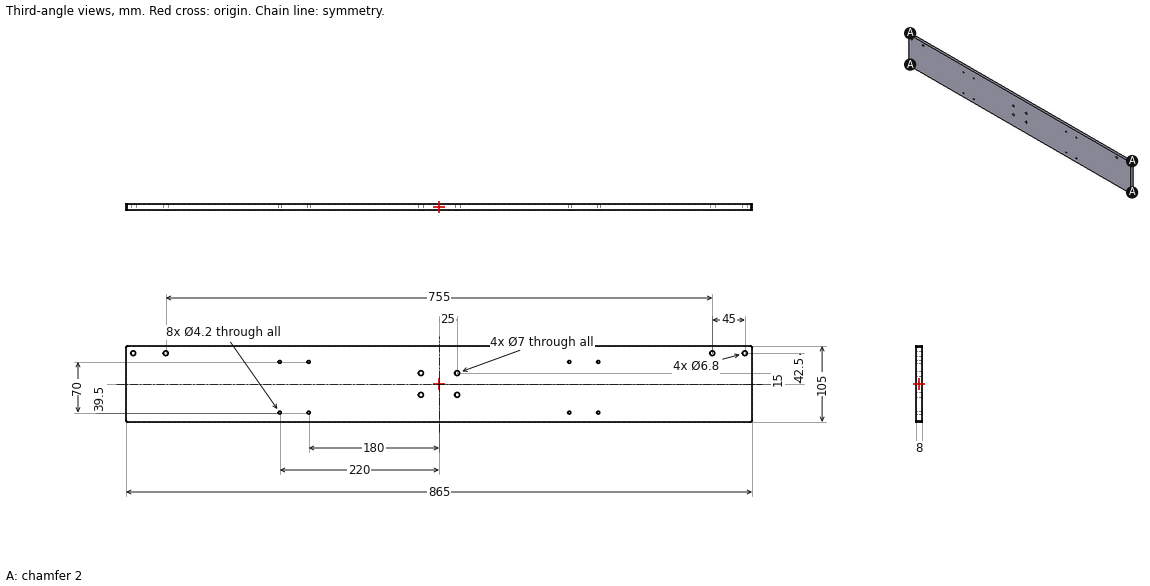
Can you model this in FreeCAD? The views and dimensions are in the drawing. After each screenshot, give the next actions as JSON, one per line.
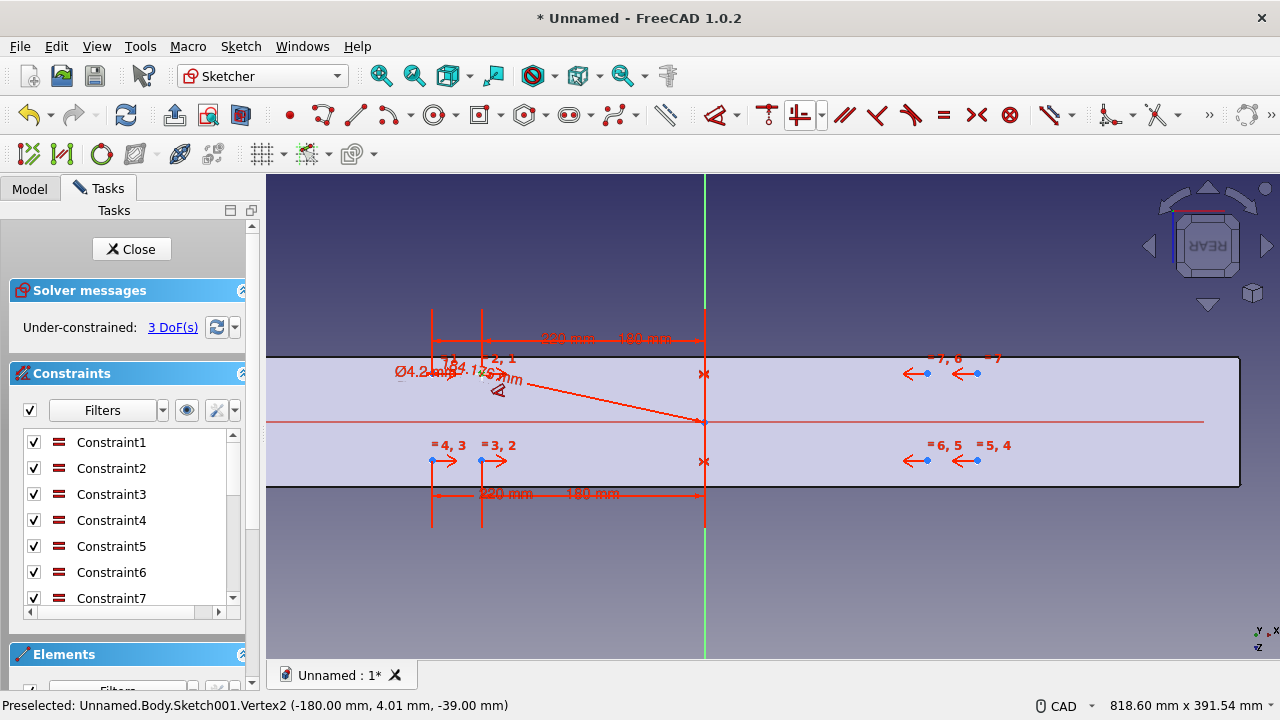
{"action": "left_click", "coordinate": [482, 461]}
{"action": "left_click", "coordinate": [448, 397]}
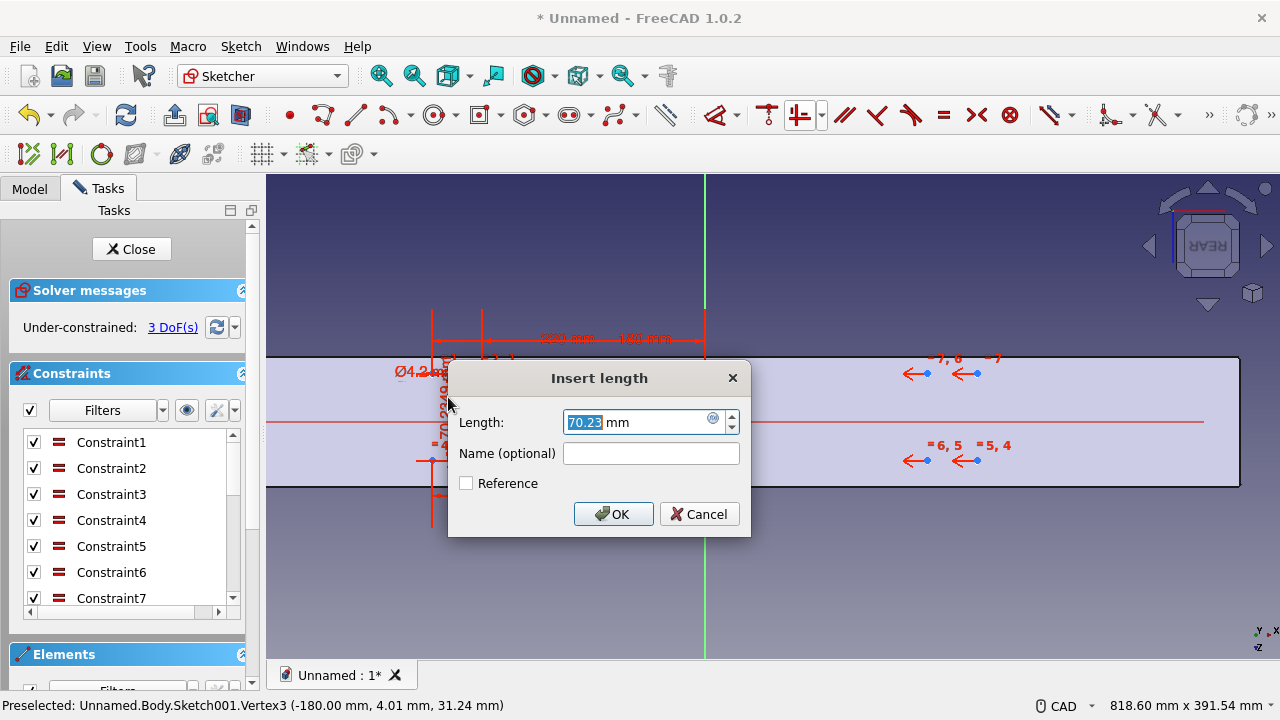
{"action": "type", "text": "70"}
{"action": "key", "text": "Return"}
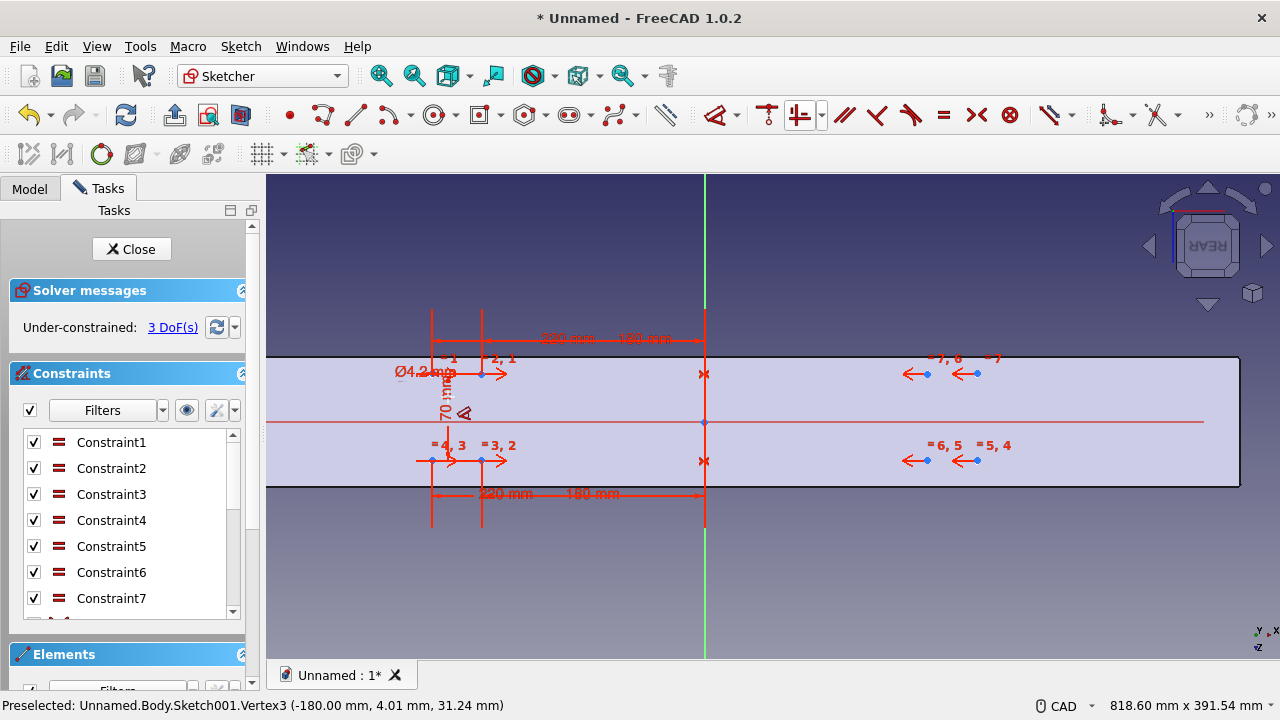
{"action": "left_click", "coordinate": [432, 374]}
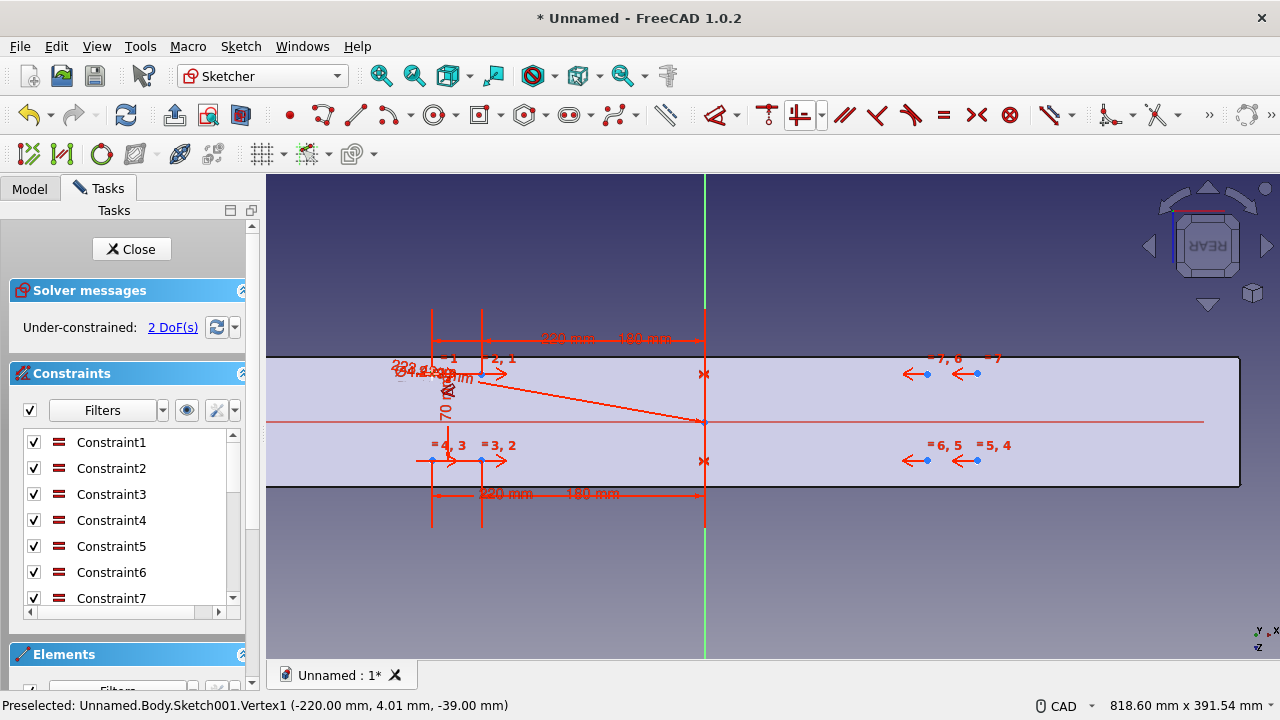
{"action": "left_click", "coordinate": [482, 461]}
{"action": "left_click", "coordinate": [398, 437]}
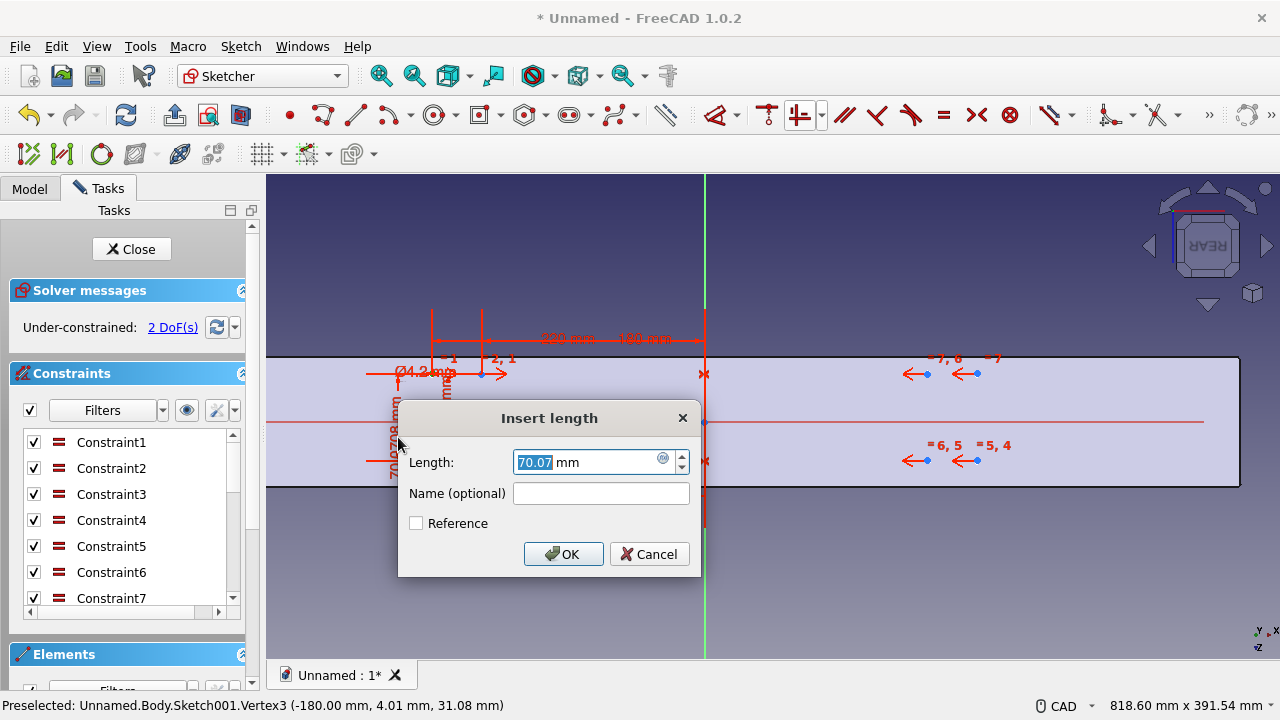
{"action": "type", "text": "70"}
{"action": "key", "text": "Return"}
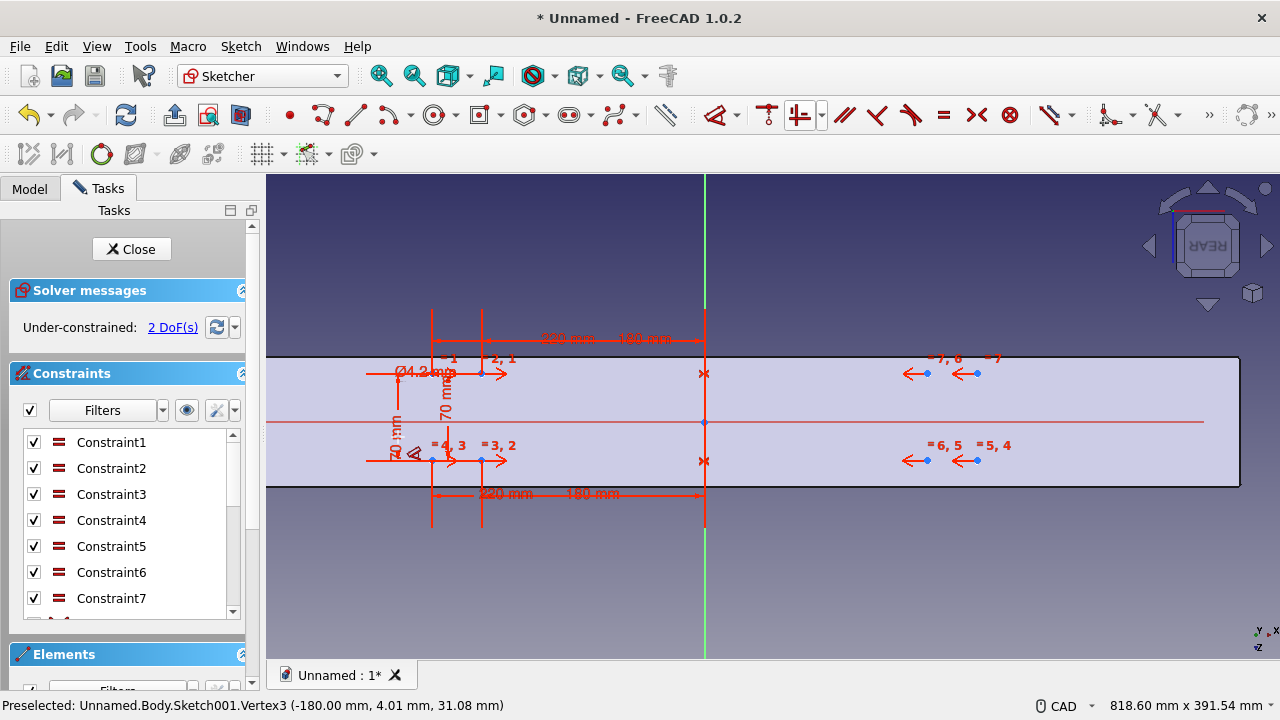
{"action": "left_click", "coordinate": [432, 374]}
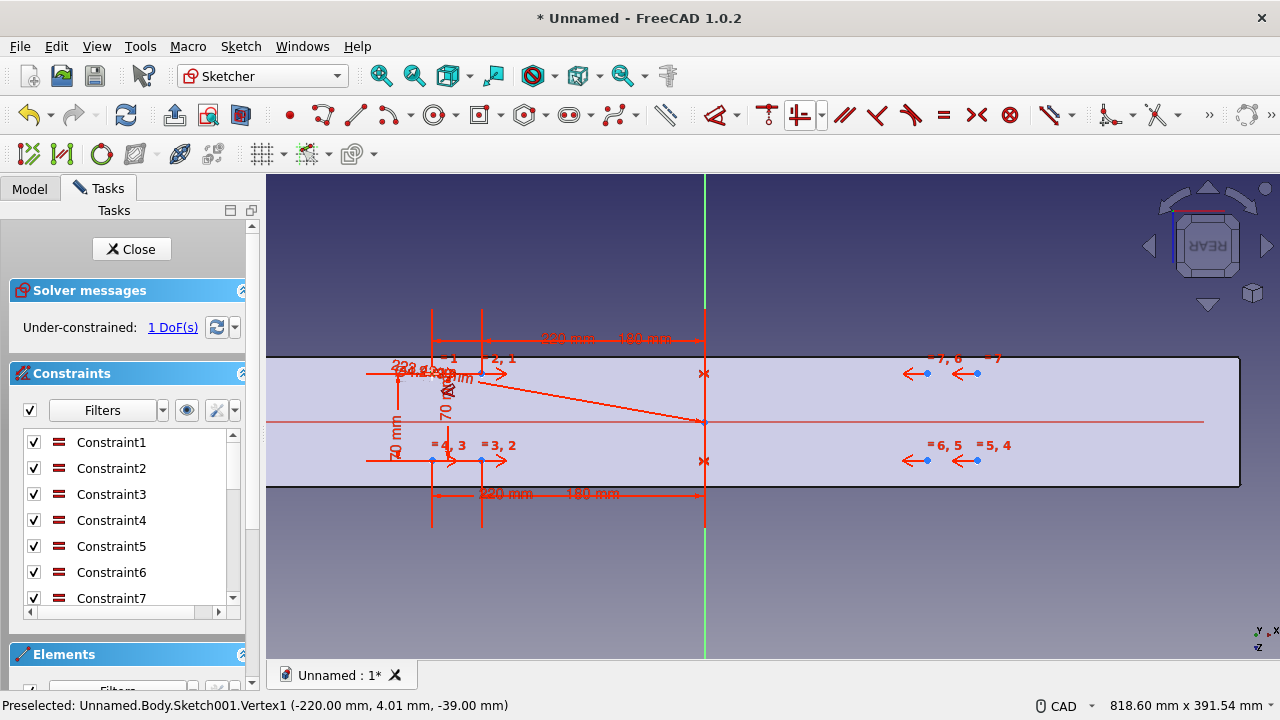
{"action": "left_click", "coordinate": [432, 461]}
{"action": "left_click", "coordinate": [374, 397]}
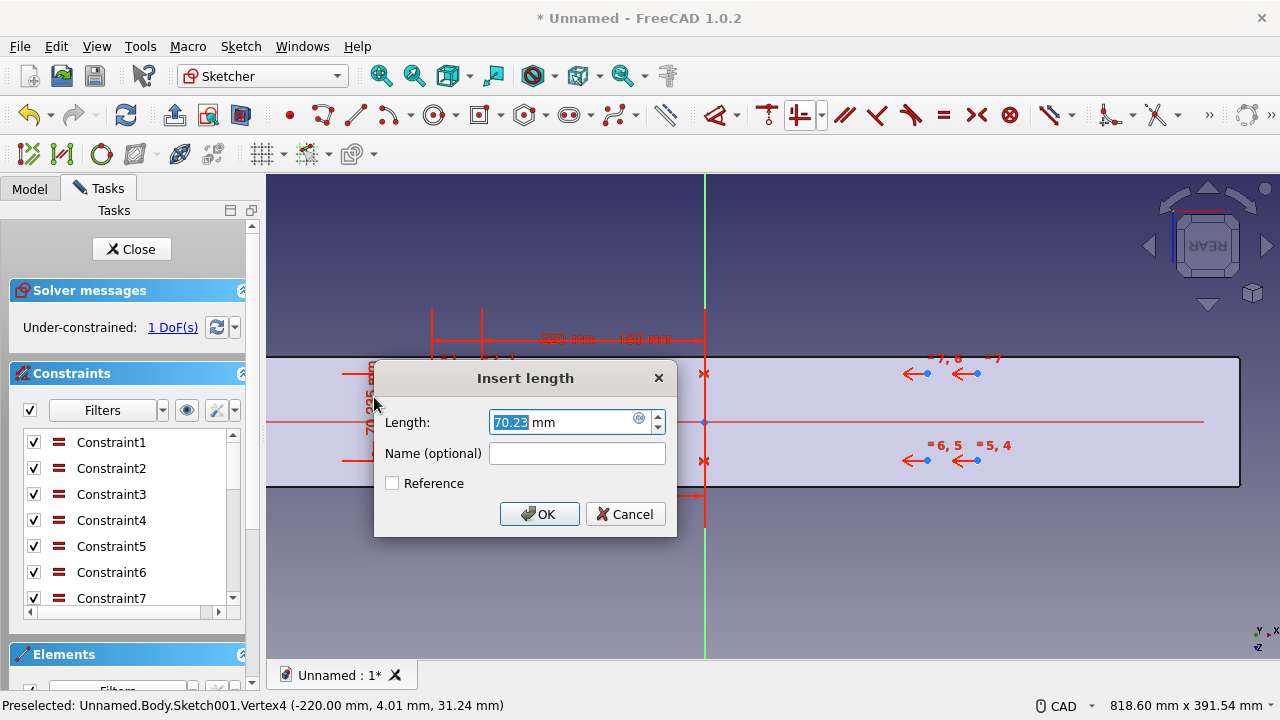
{"action": "type", "text": "70"}
{"action": "key", "text": "Return"}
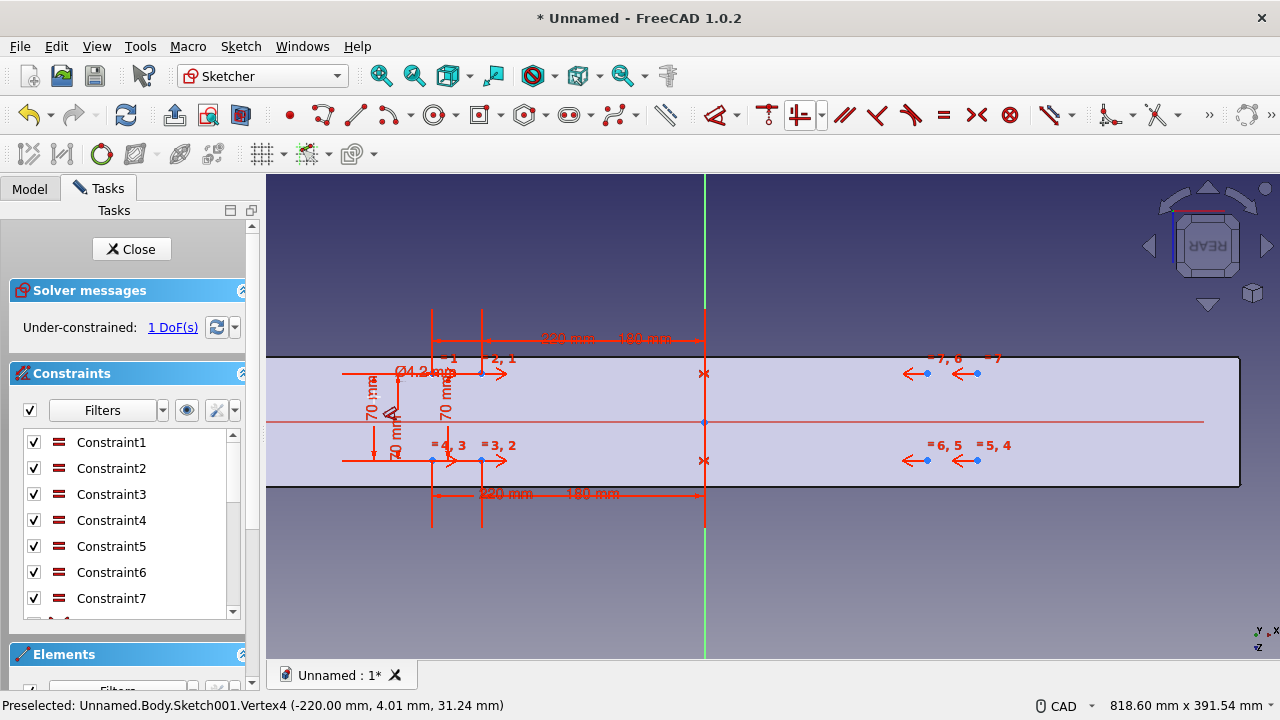
{"action": "left_click", "coordinate": [432, 374]}
{"action": "left_click", "coordinate": [739, 398]}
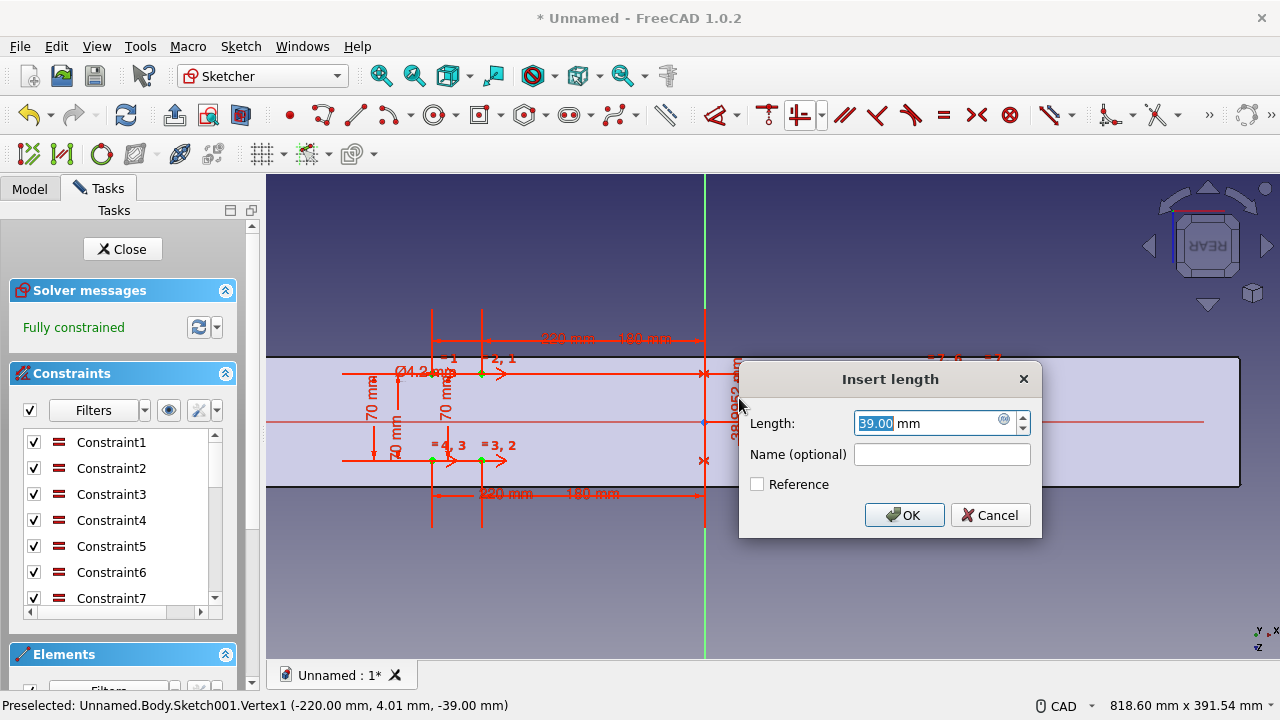
{"action": "type", "text": "39.5"}
{"action": "key", "text": "Return"}
{"action": "key", "text": "Escape"}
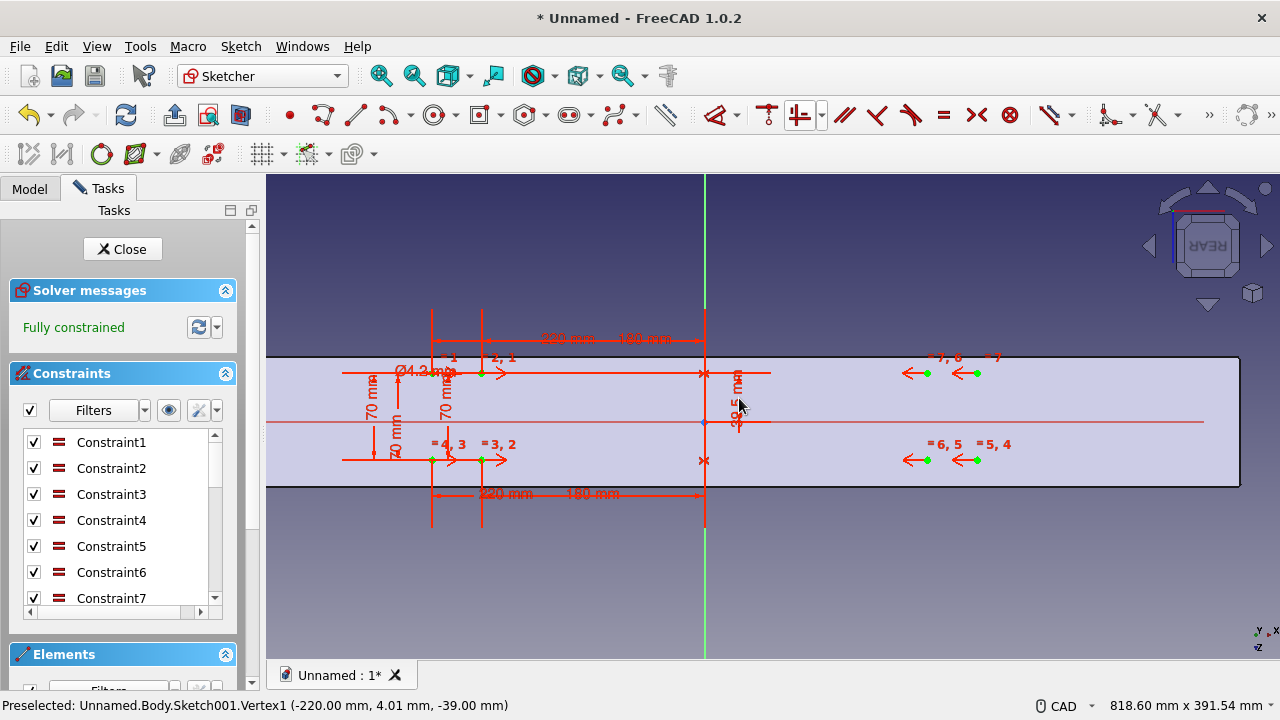
{"action": "left_click", "coordinate": [123, 249]}